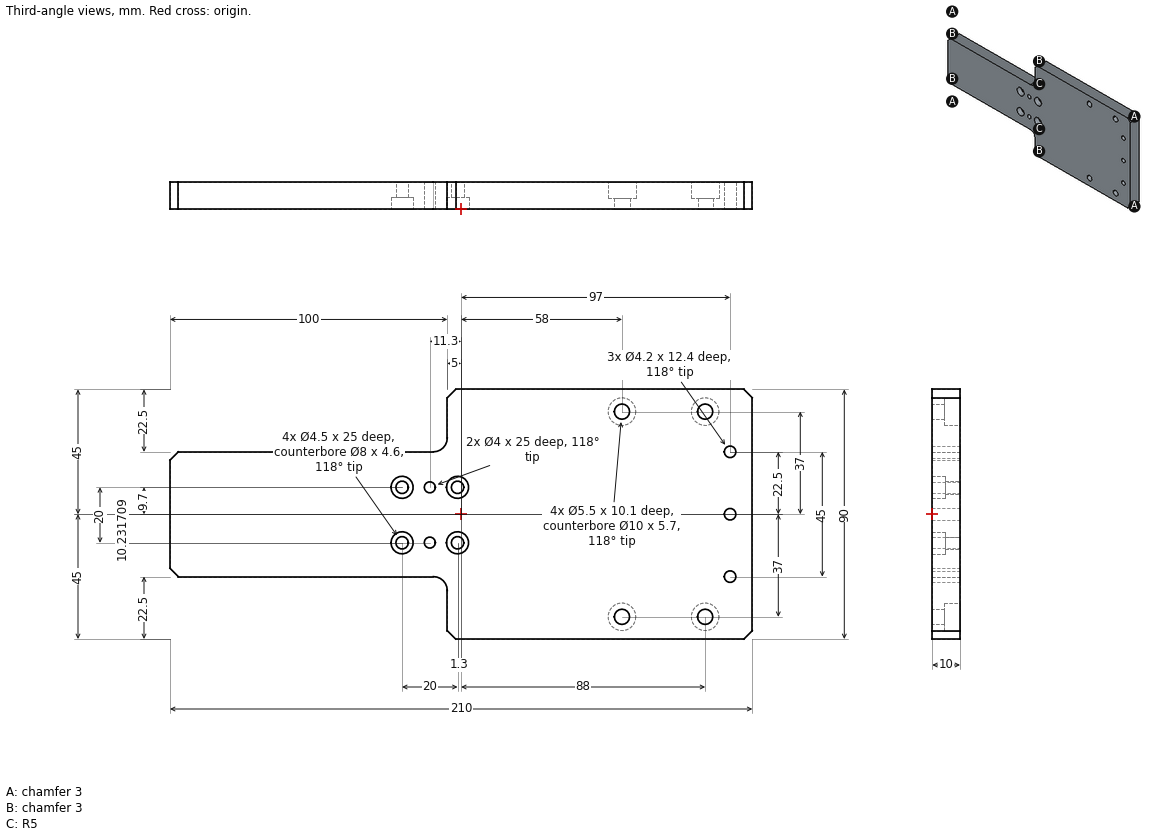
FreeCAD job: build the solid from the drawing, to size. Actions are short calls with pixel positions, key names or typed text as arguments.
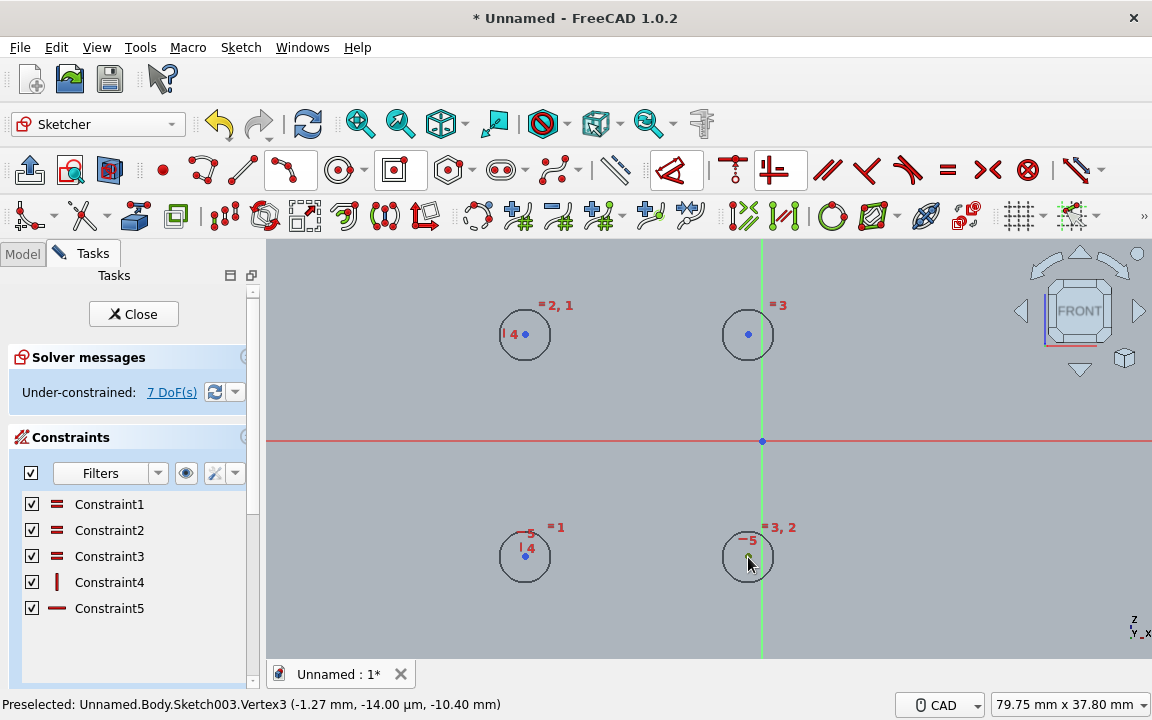
click(748, 335)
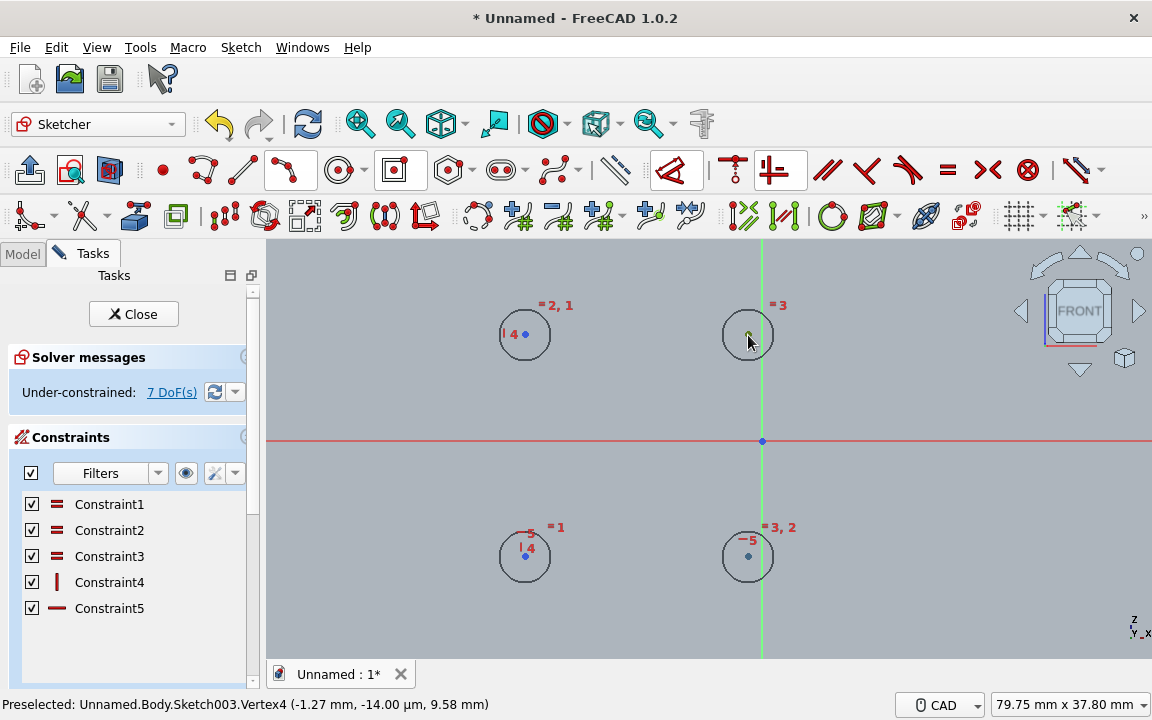
key(v)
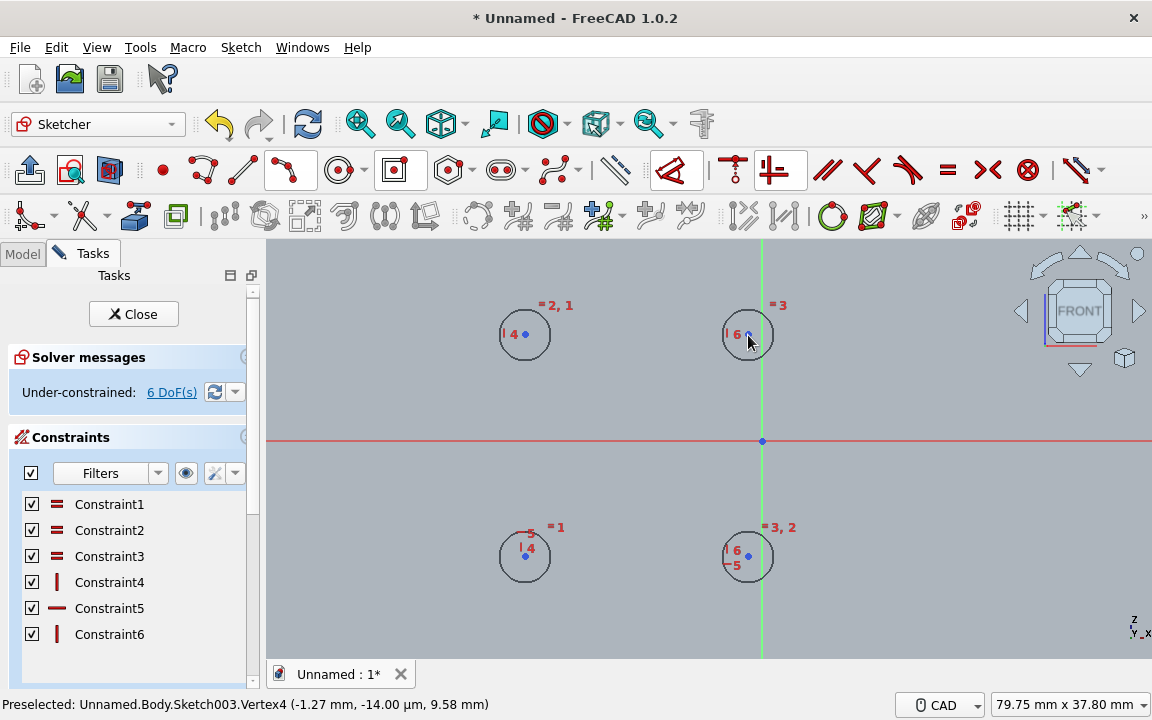
click(525, 335)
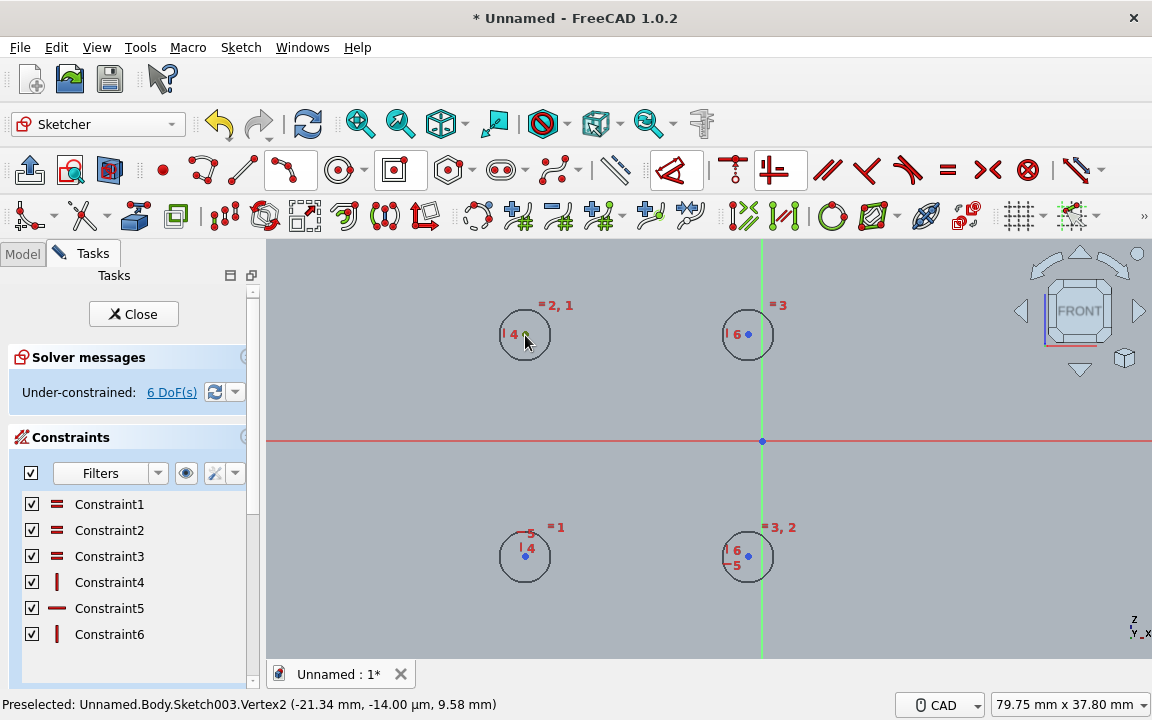
click(748, 335)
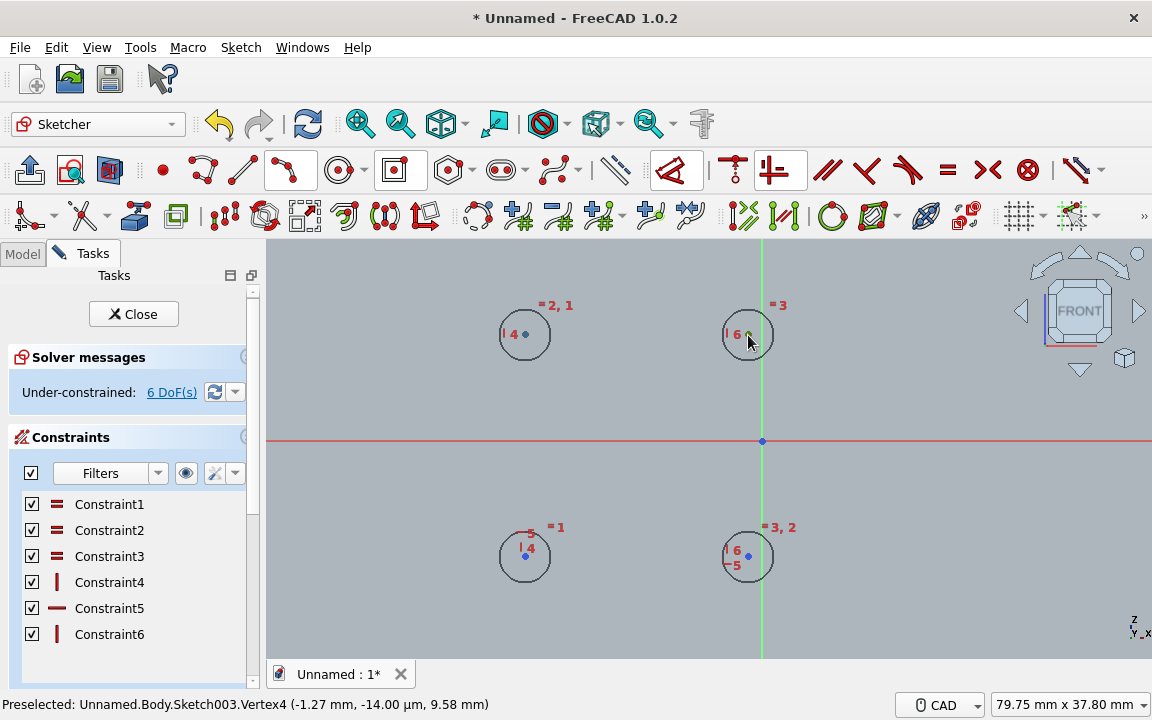
click(802, 170)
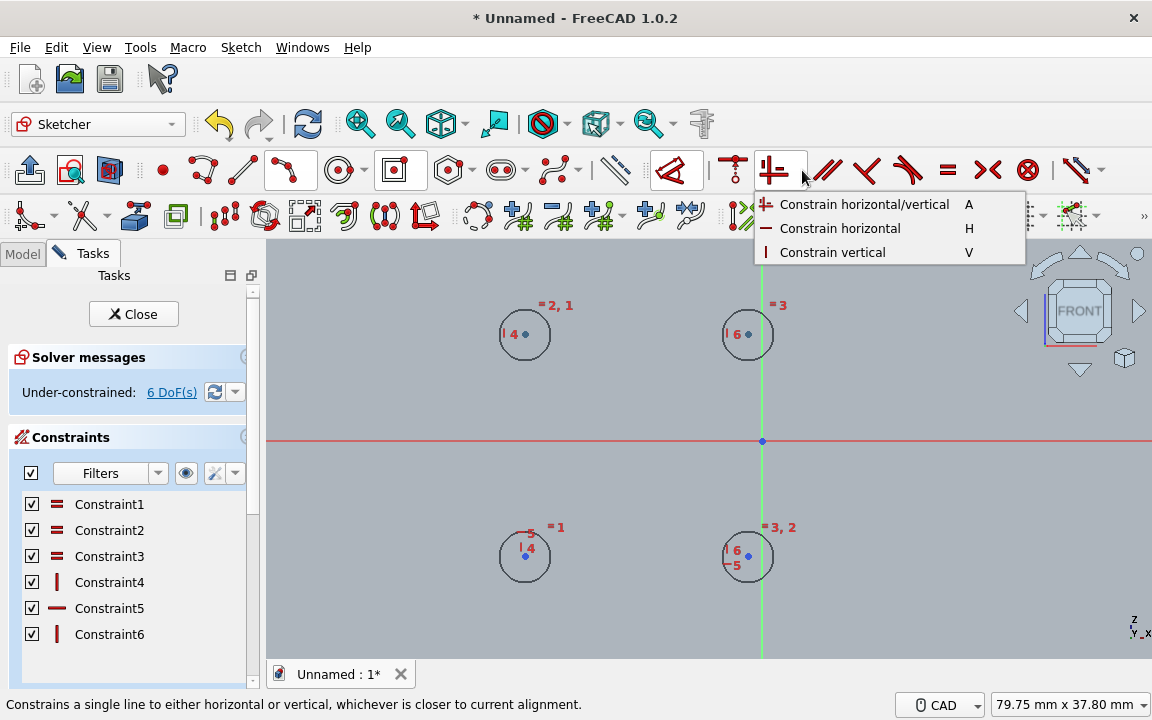
click(890, 228)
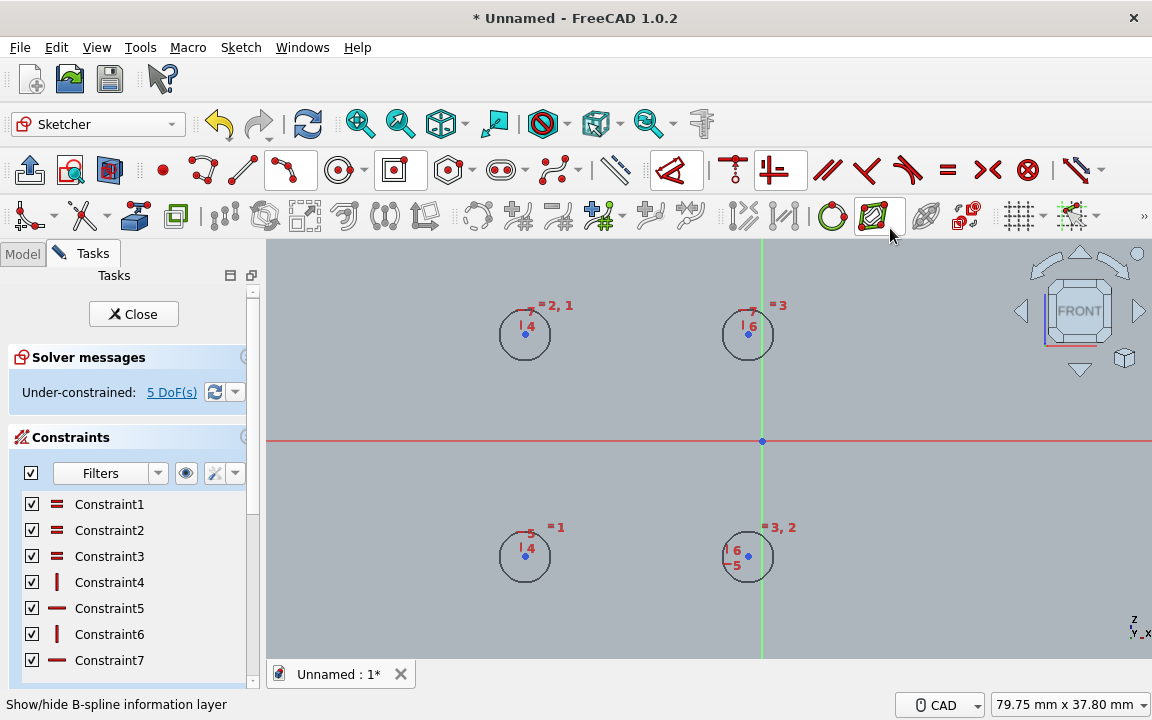
click(543, 539)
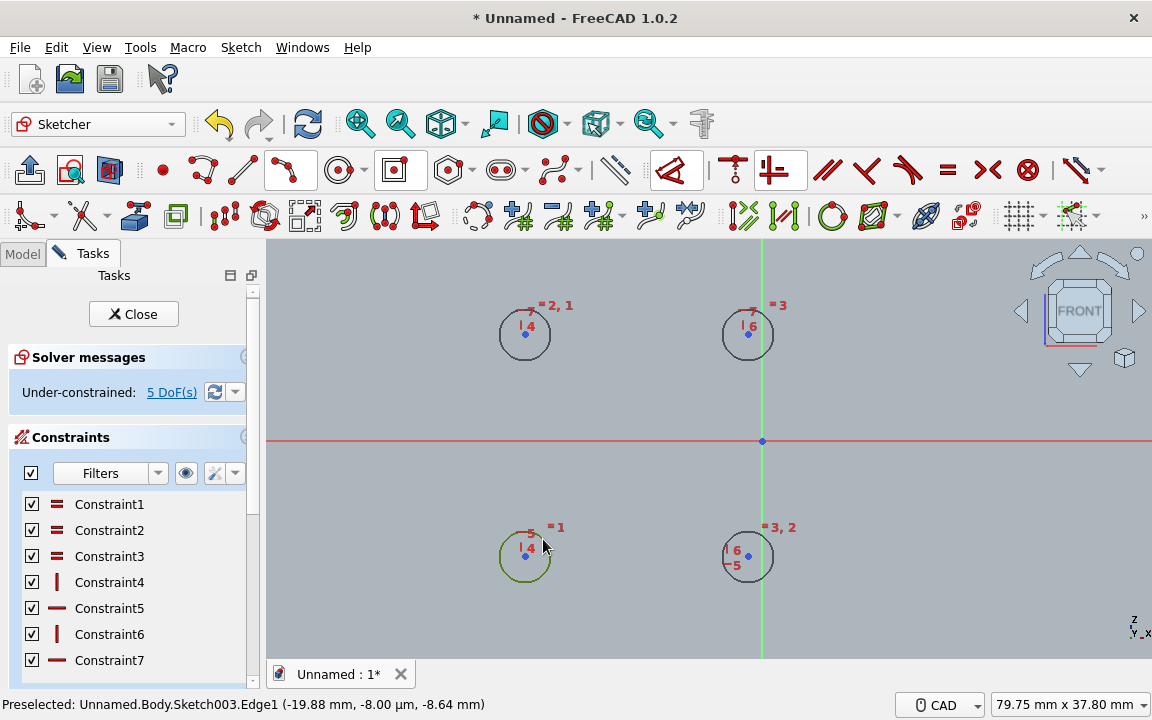
click(698, 170)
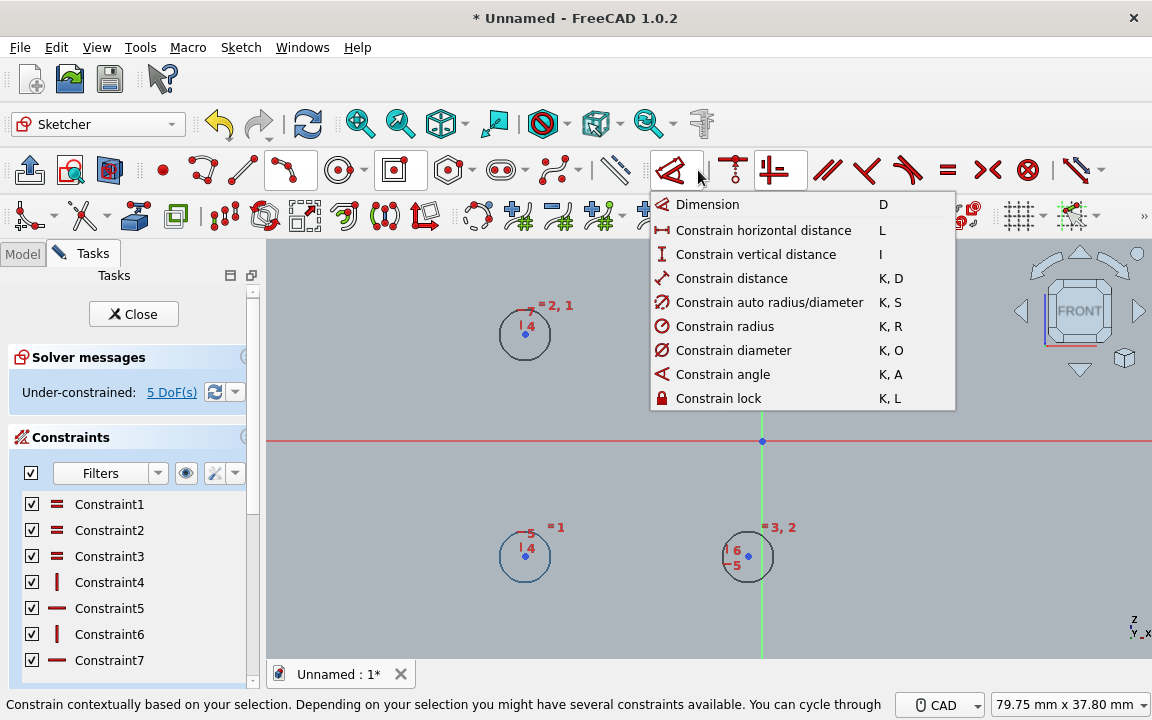
click(803, 350)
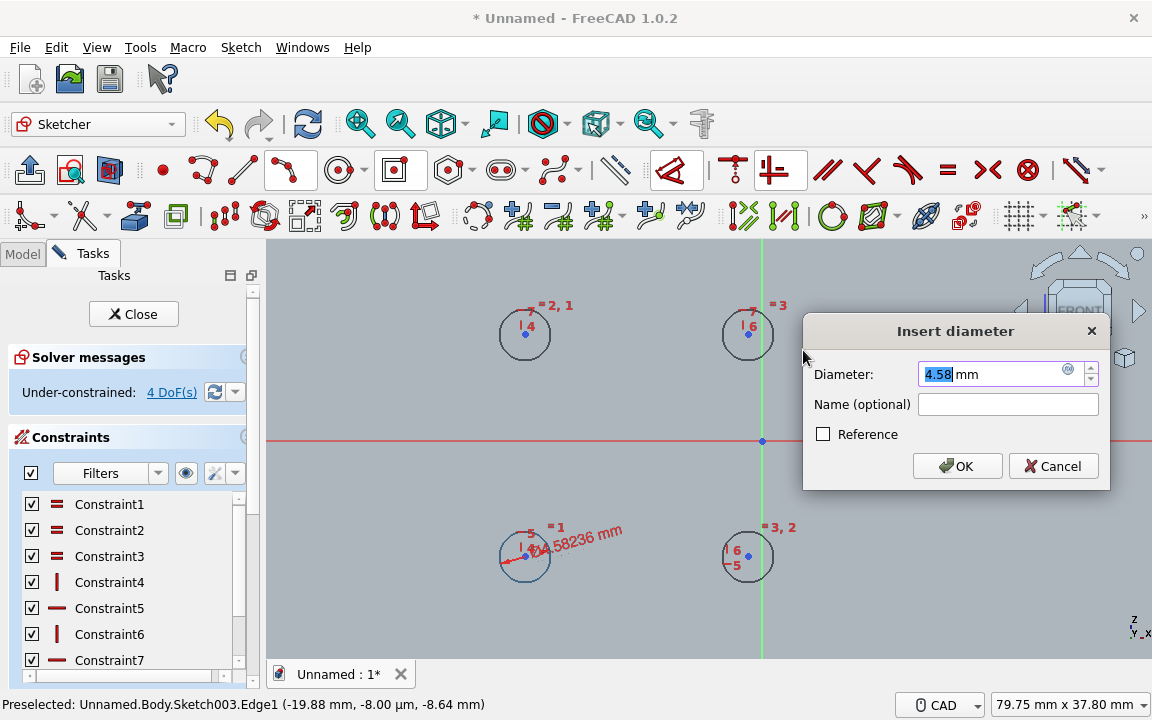
text(4.5)
key(Return)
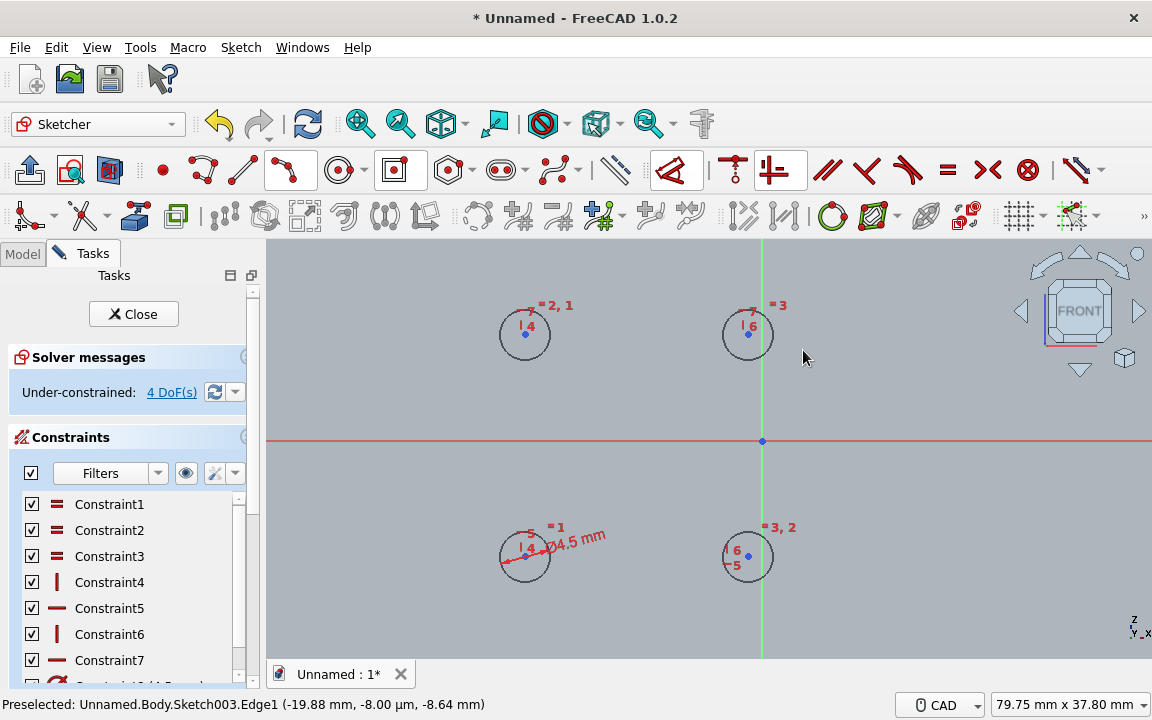
click(525, 335)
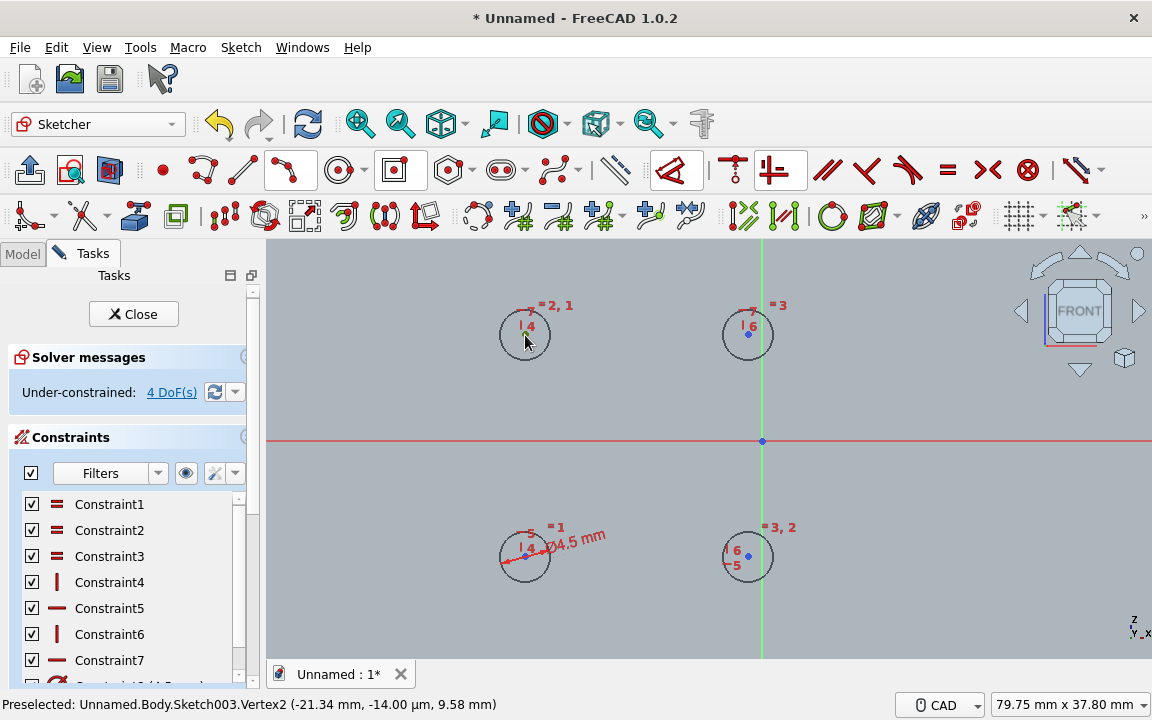
click(698, 170)